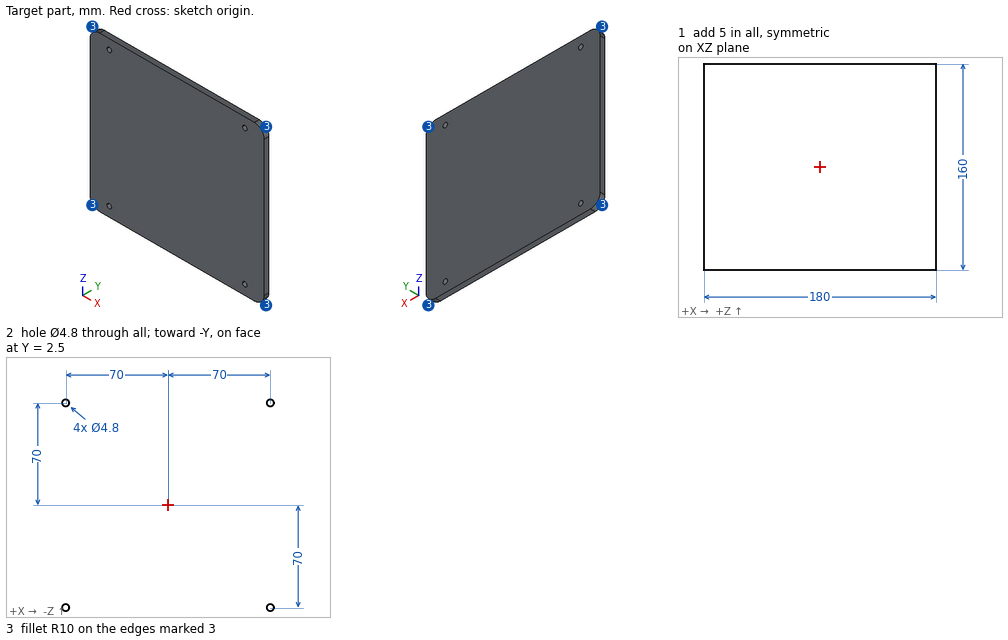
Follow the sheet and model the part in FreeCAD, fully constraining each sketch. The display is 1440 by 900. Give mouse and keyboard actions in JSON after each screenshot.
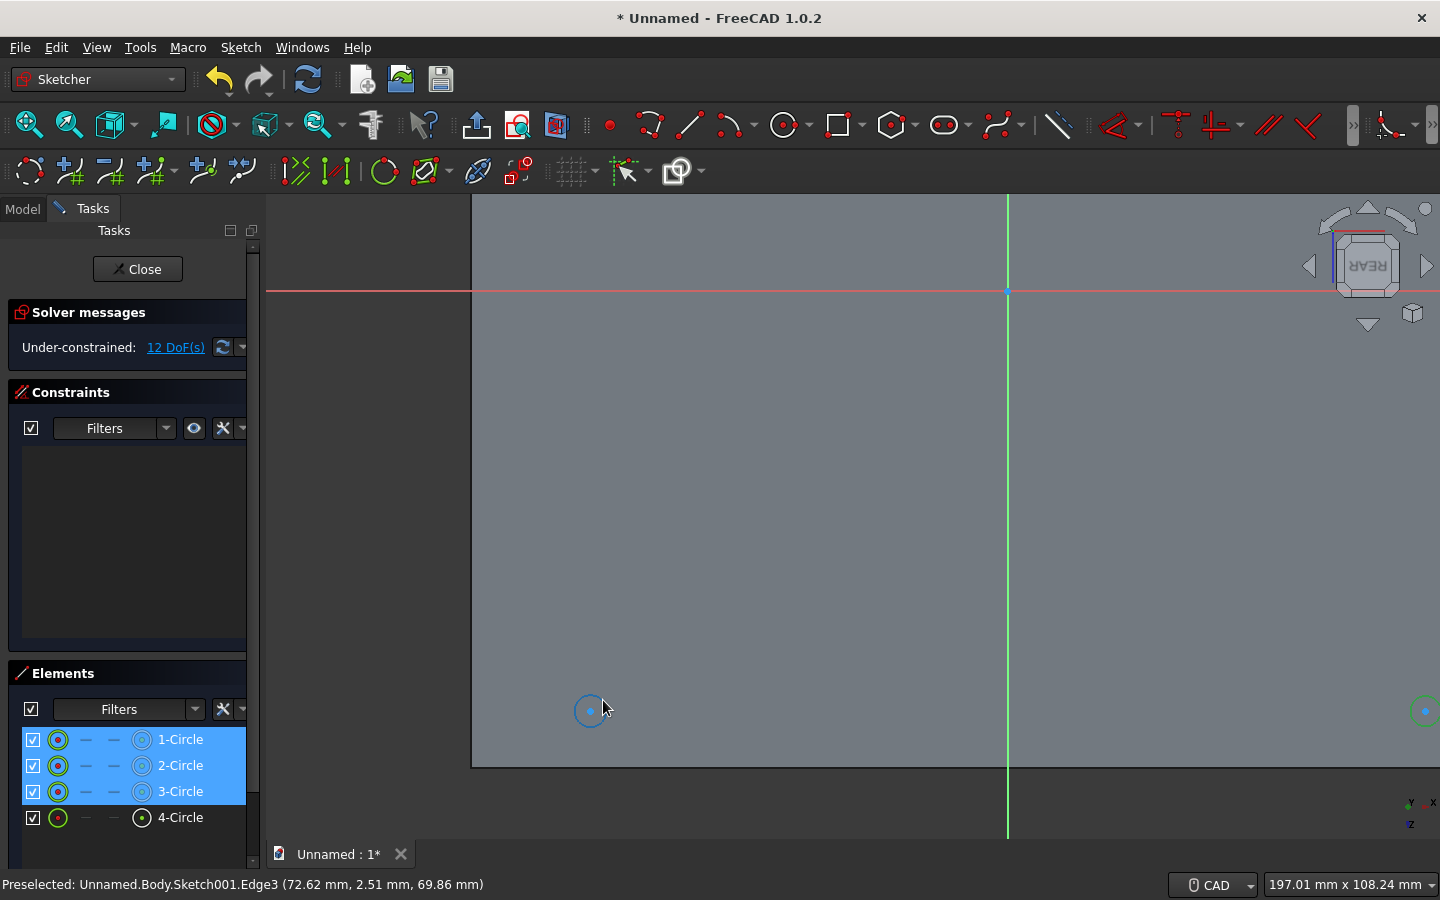
{"action": "left_click", "coordinate": [602, 700]}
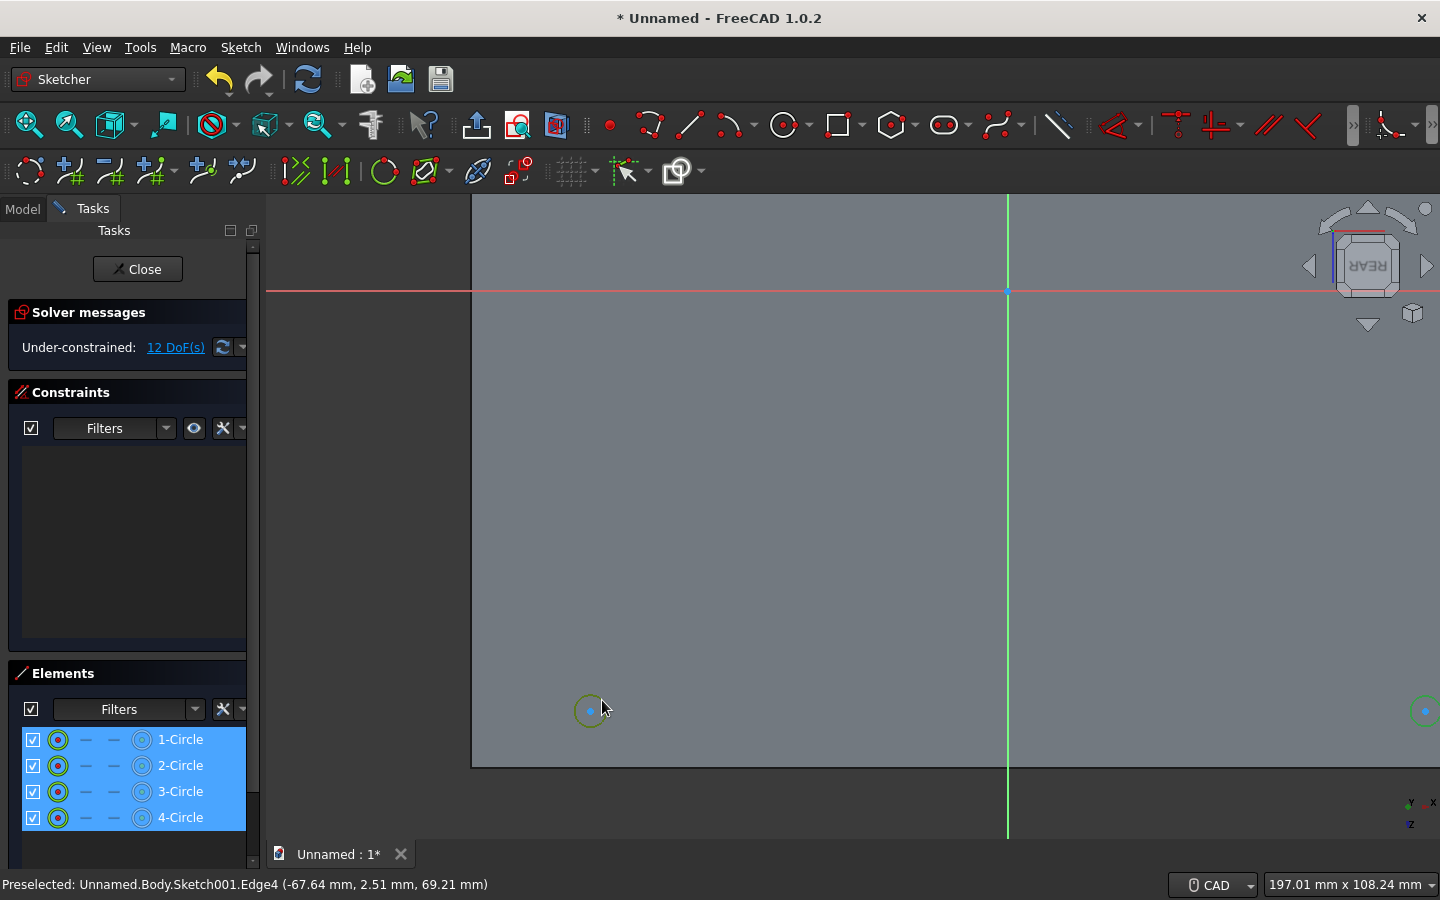
{"action": "key", "text": "e"}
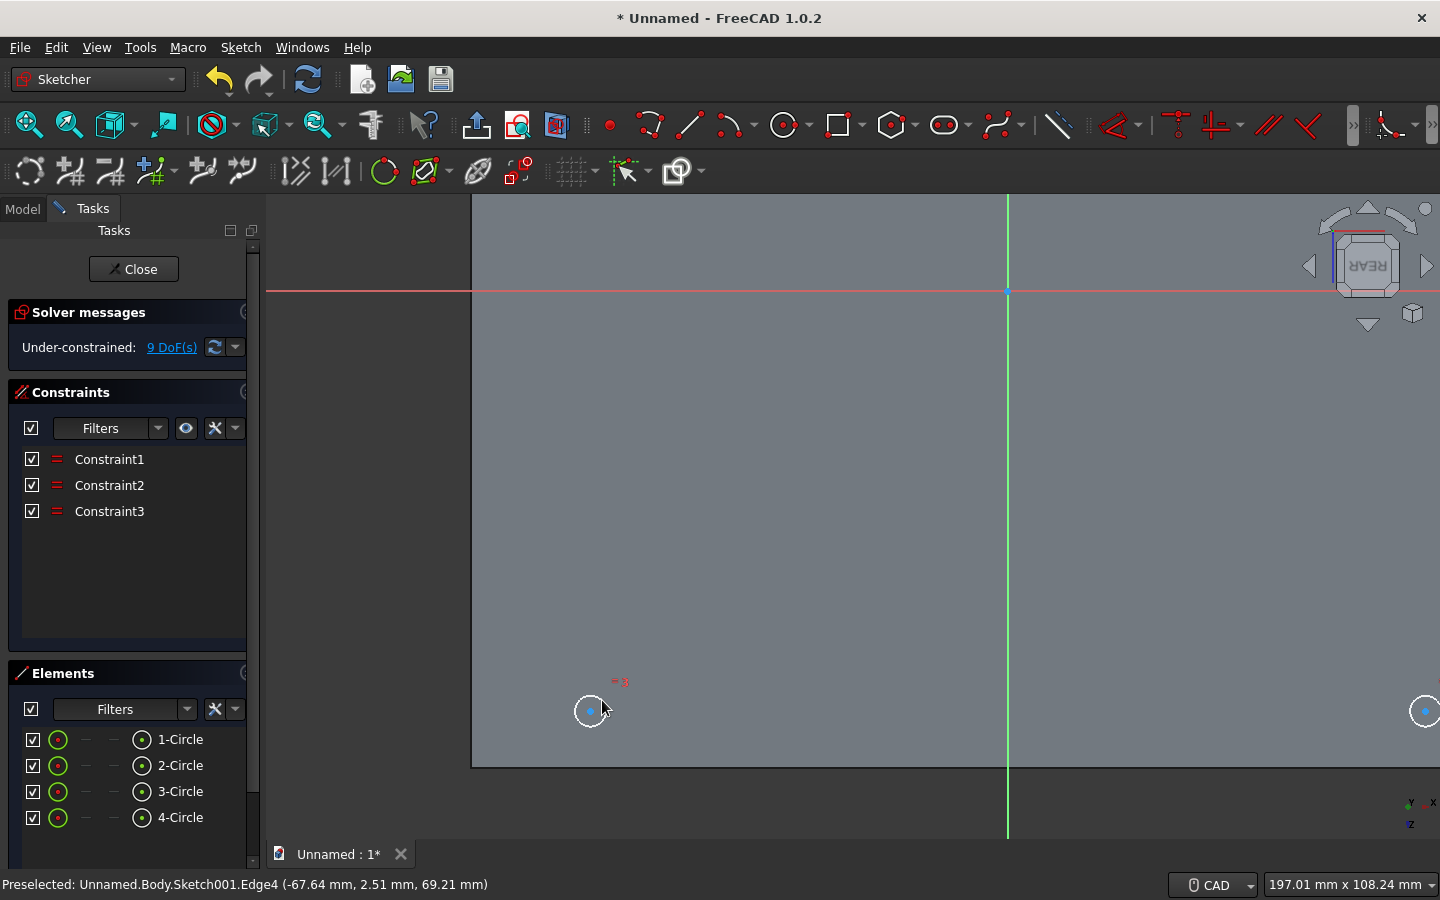
{"action": "scroll", "coordinate": [603, 700], "scroll_direction": "down", "scroll_amount": 4}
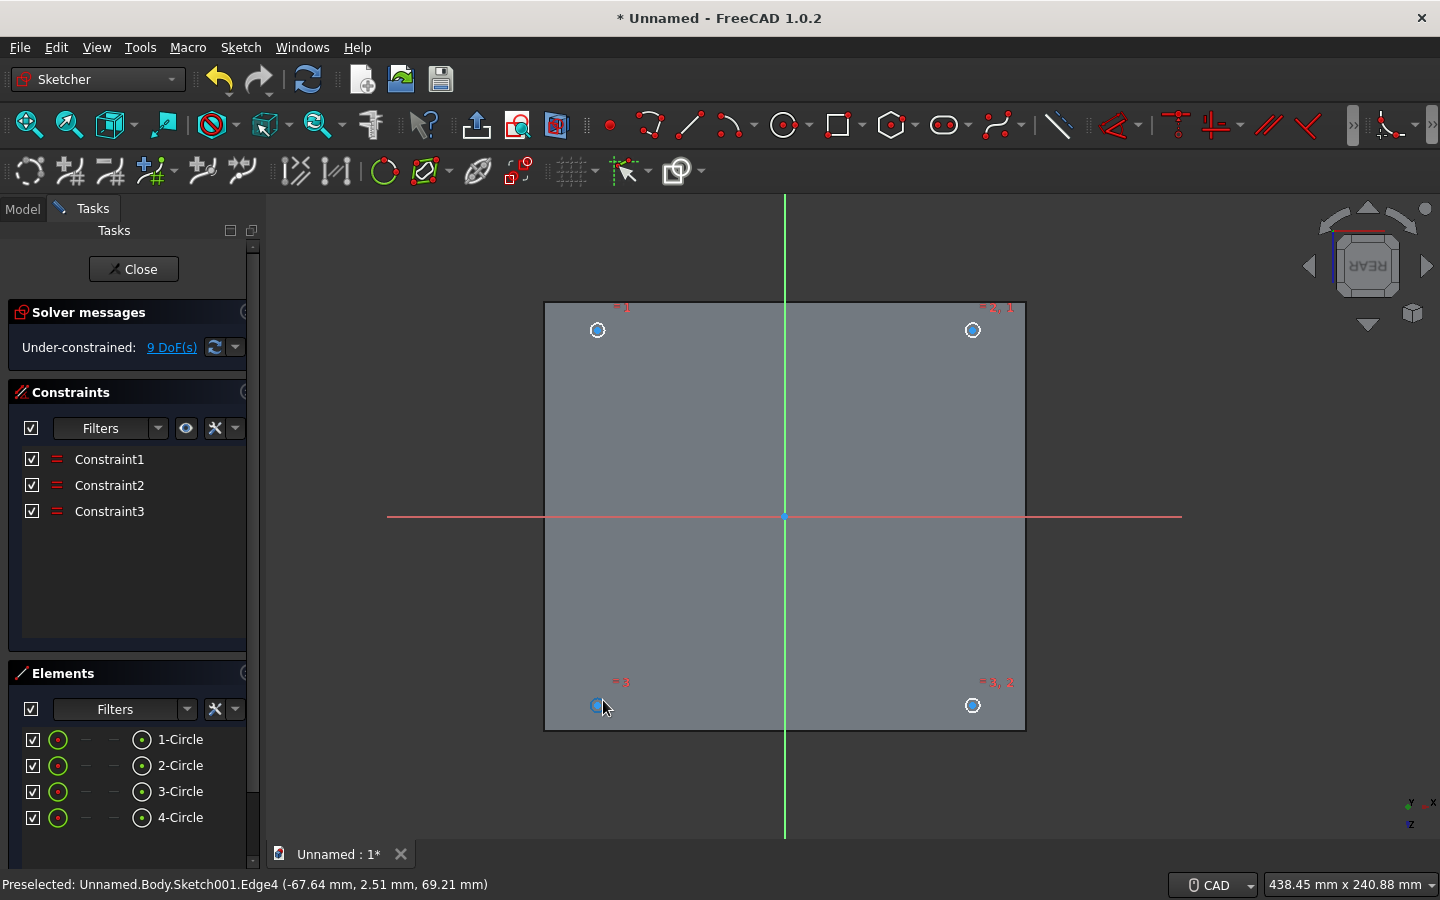
{"action": "left_click", "coordinate": [598, 330]}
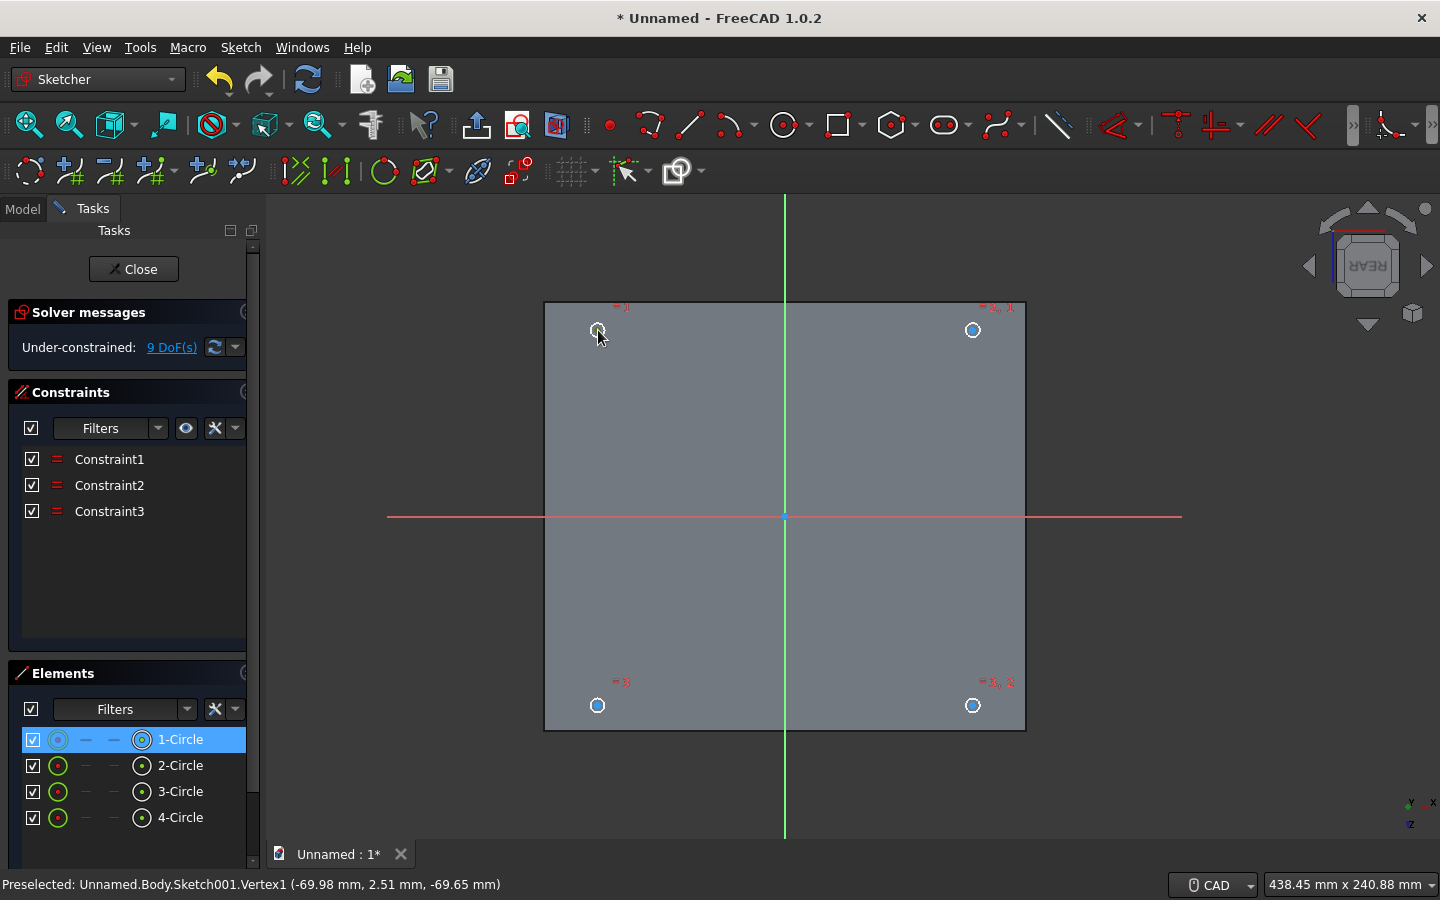
{"action": "left_click", "coordinate": [973, 330]}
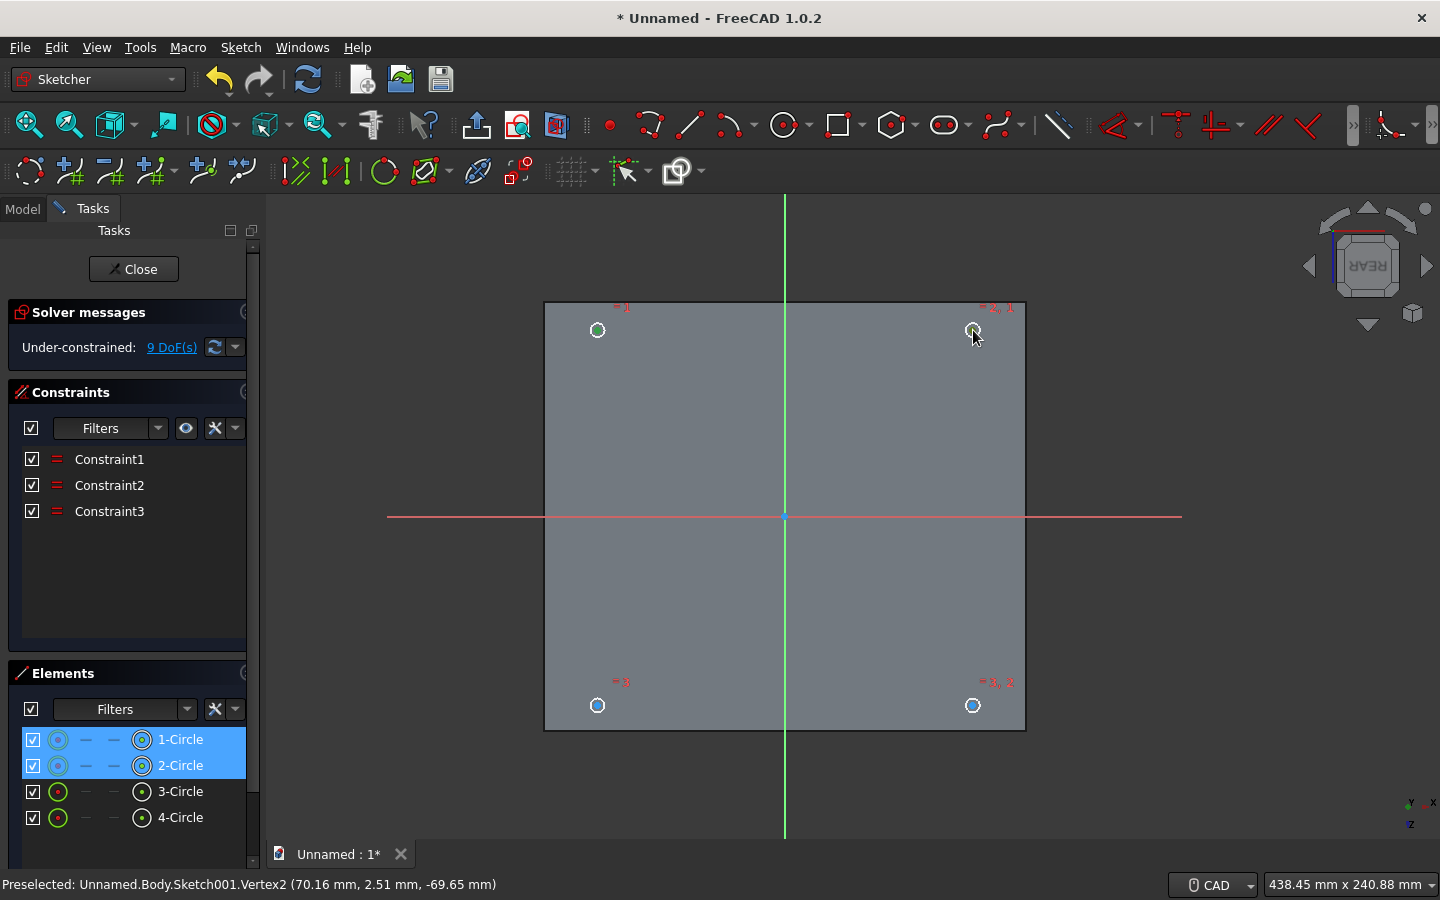
{"action": "left_click", "coordinate": [1242, 126]}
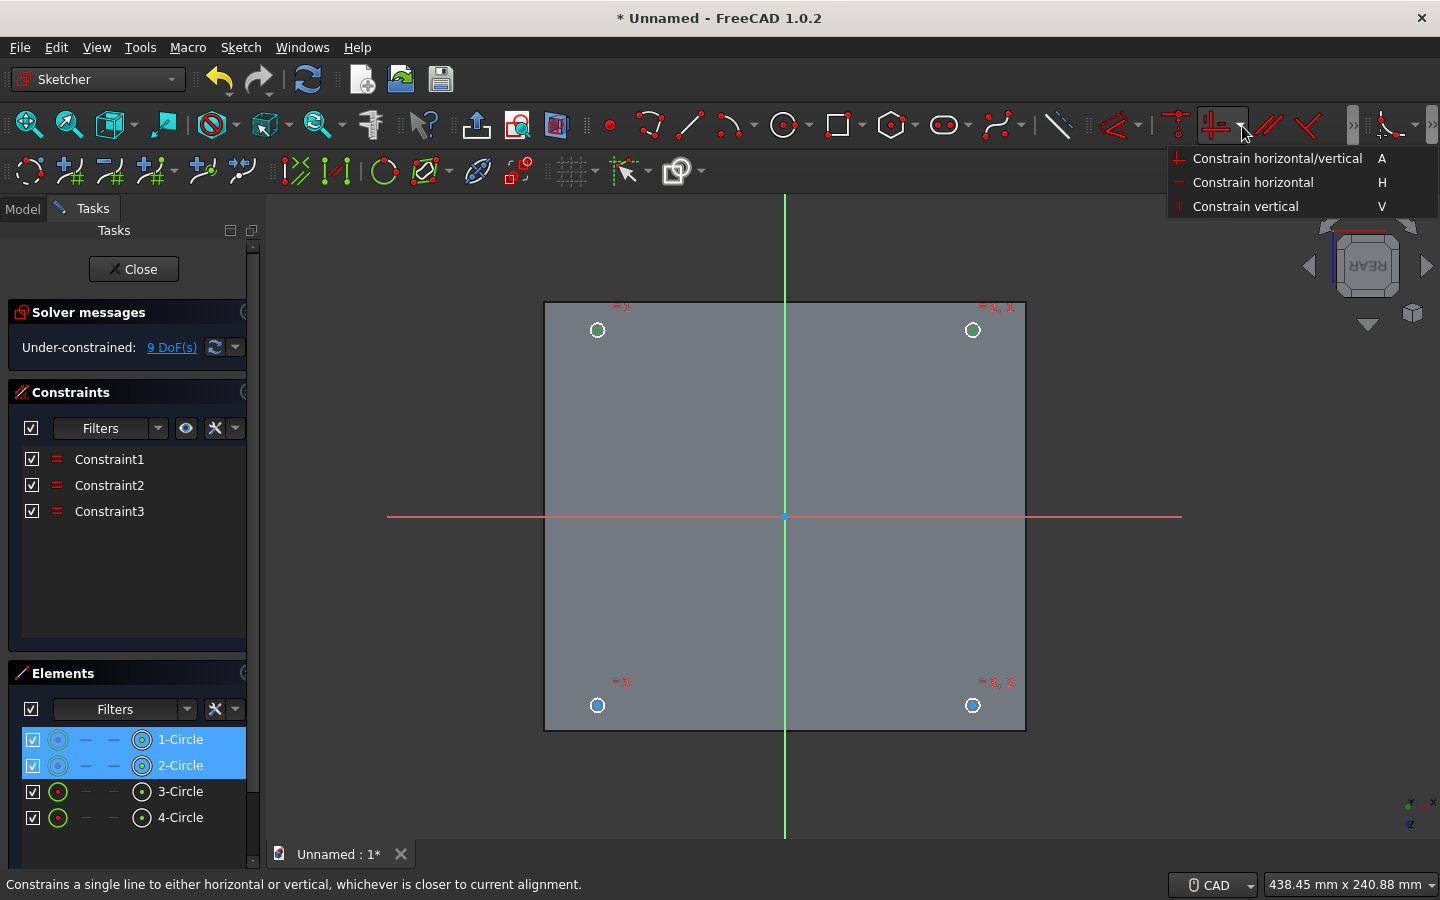
{"action": "left_click", "coordinate": [1303, 182]}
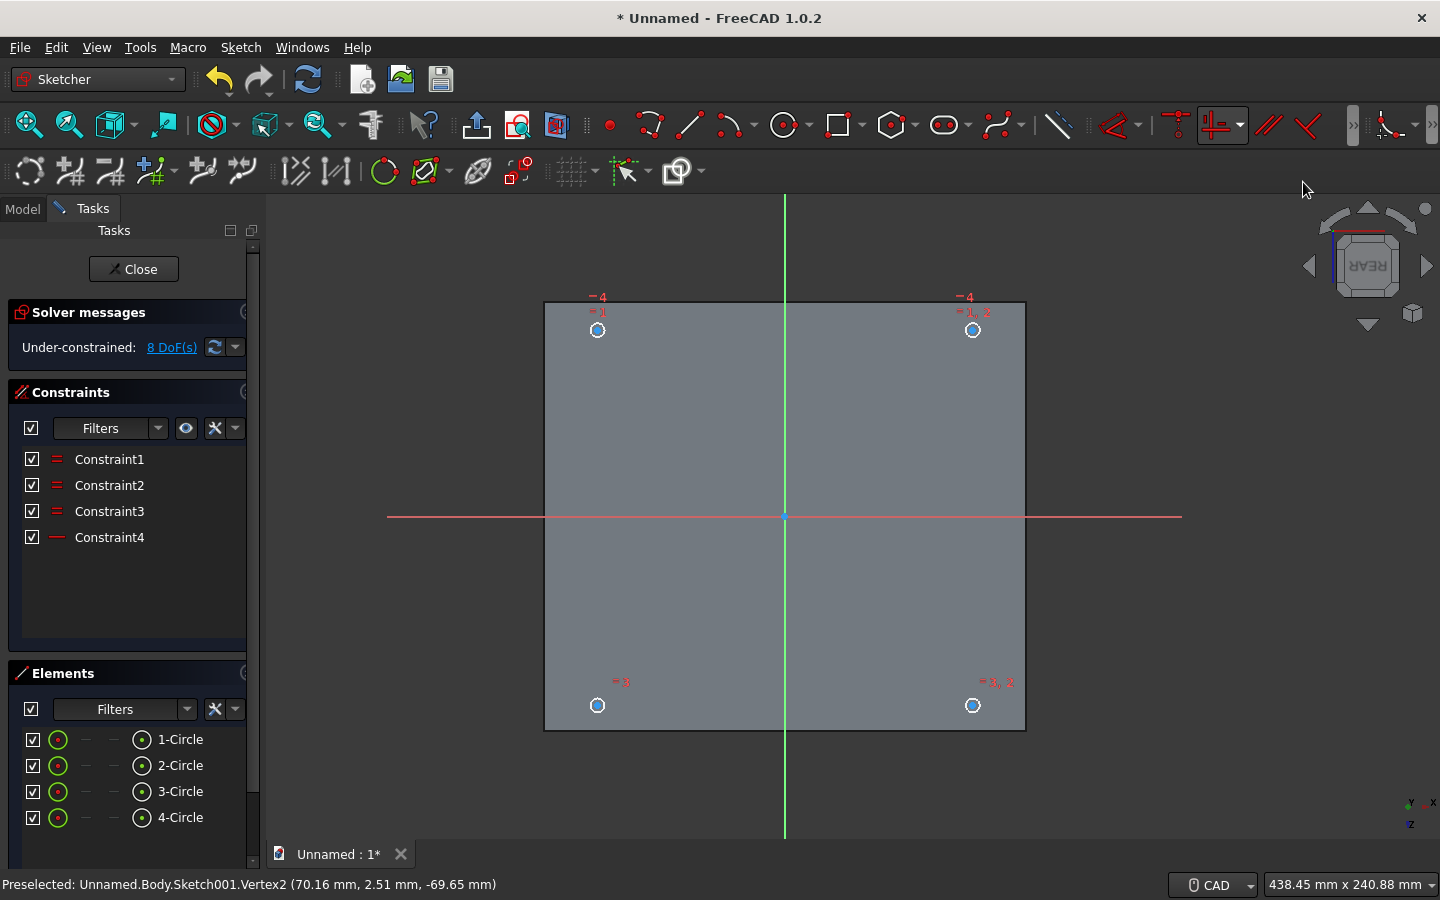
{"action": "left_click", "coordinate": [973, 330]}